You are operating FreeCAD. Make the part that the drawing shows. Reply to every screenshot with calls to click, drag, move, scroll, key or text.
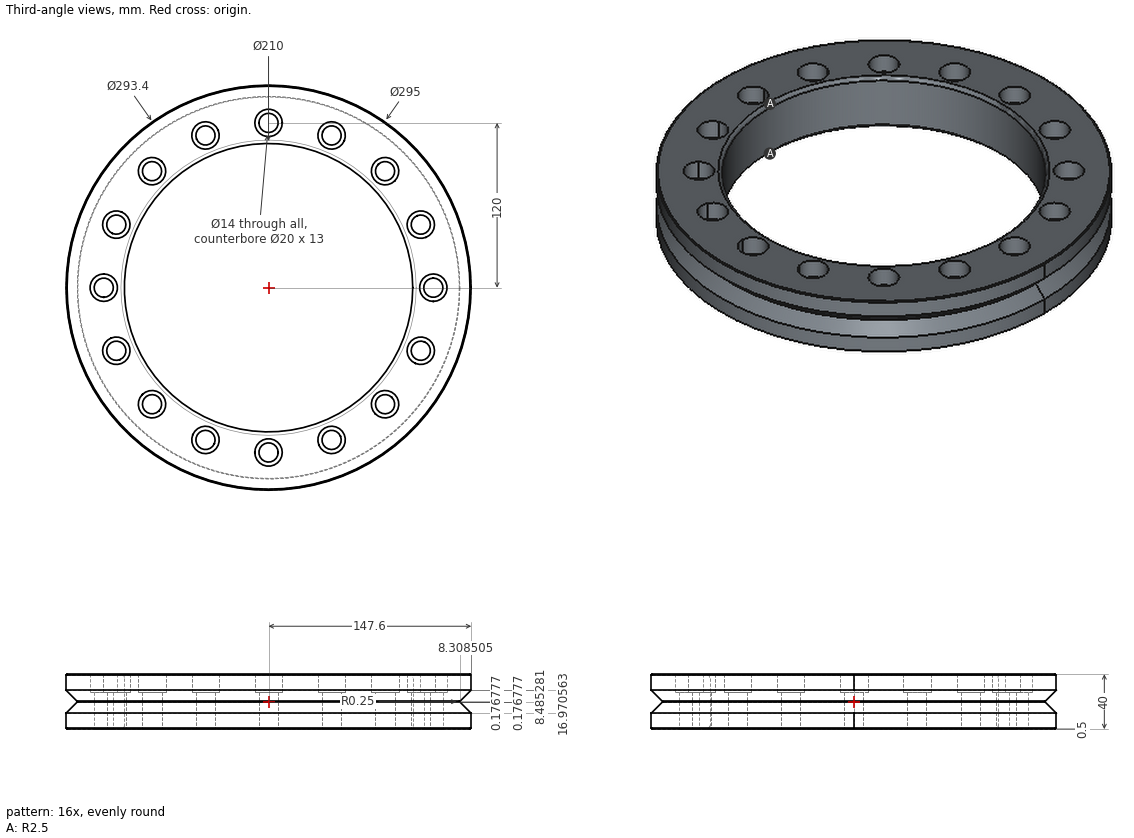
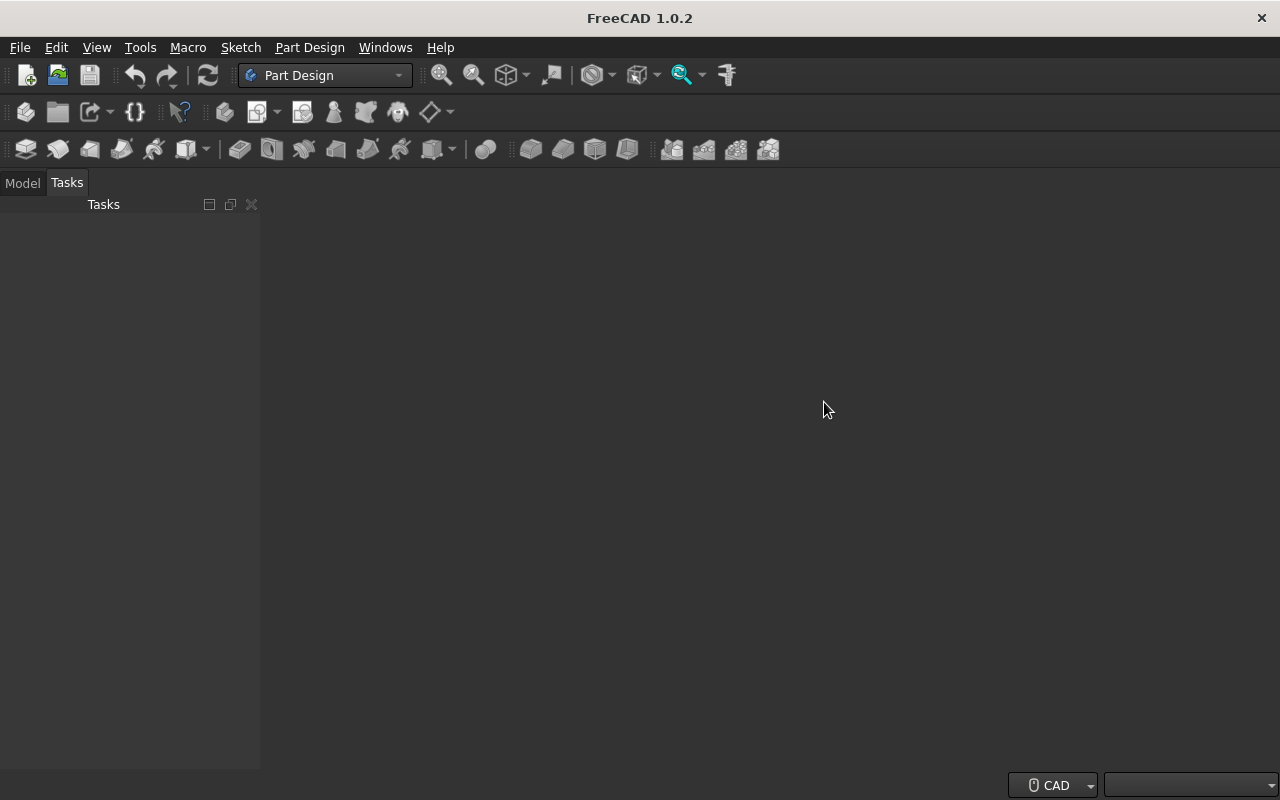
key(ctrl+n)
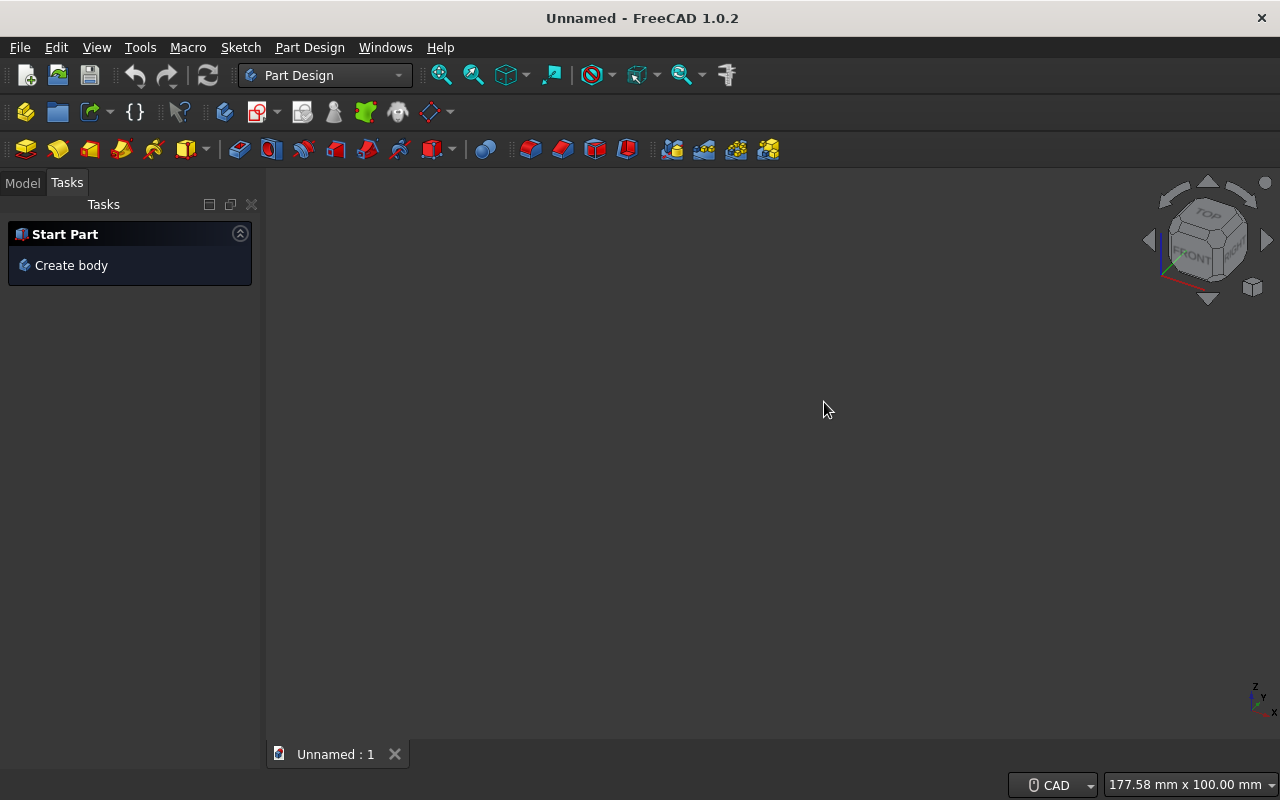
click(258, 112)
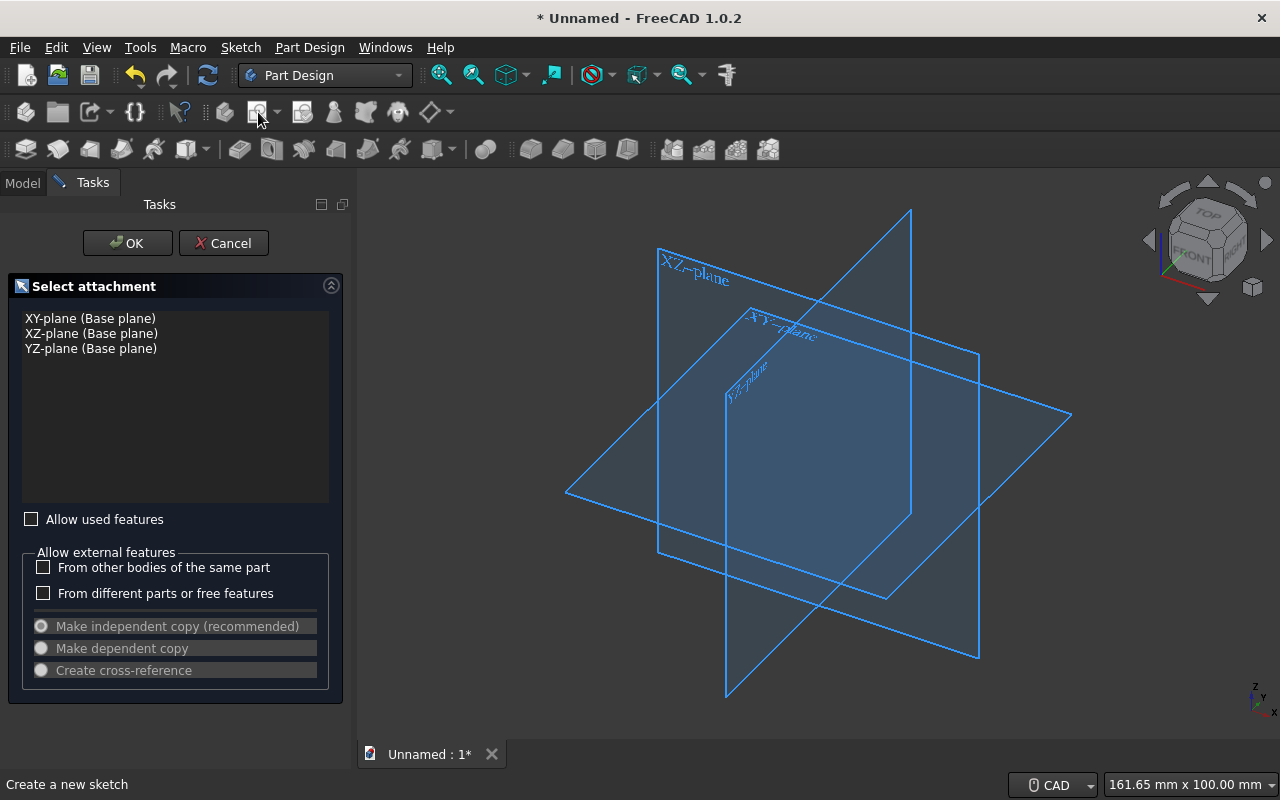
click(82, 318)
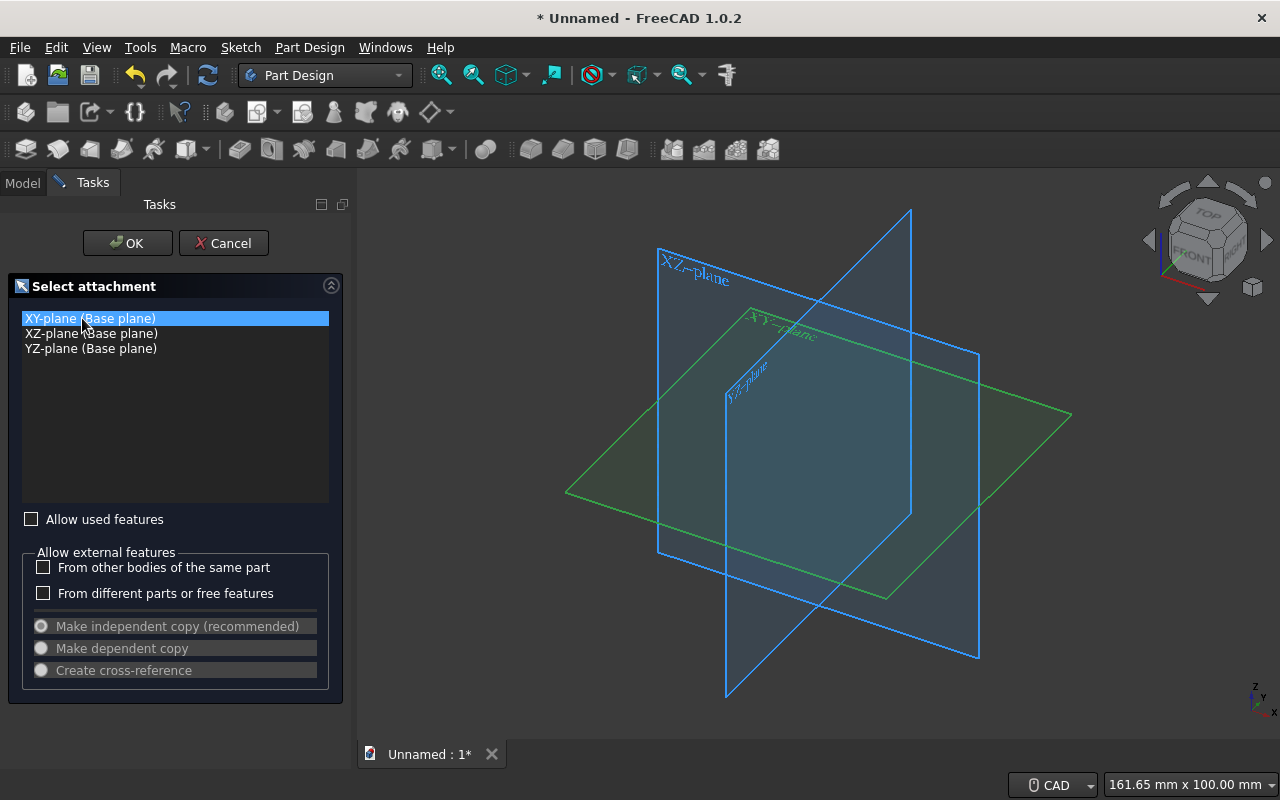
click(128, 243)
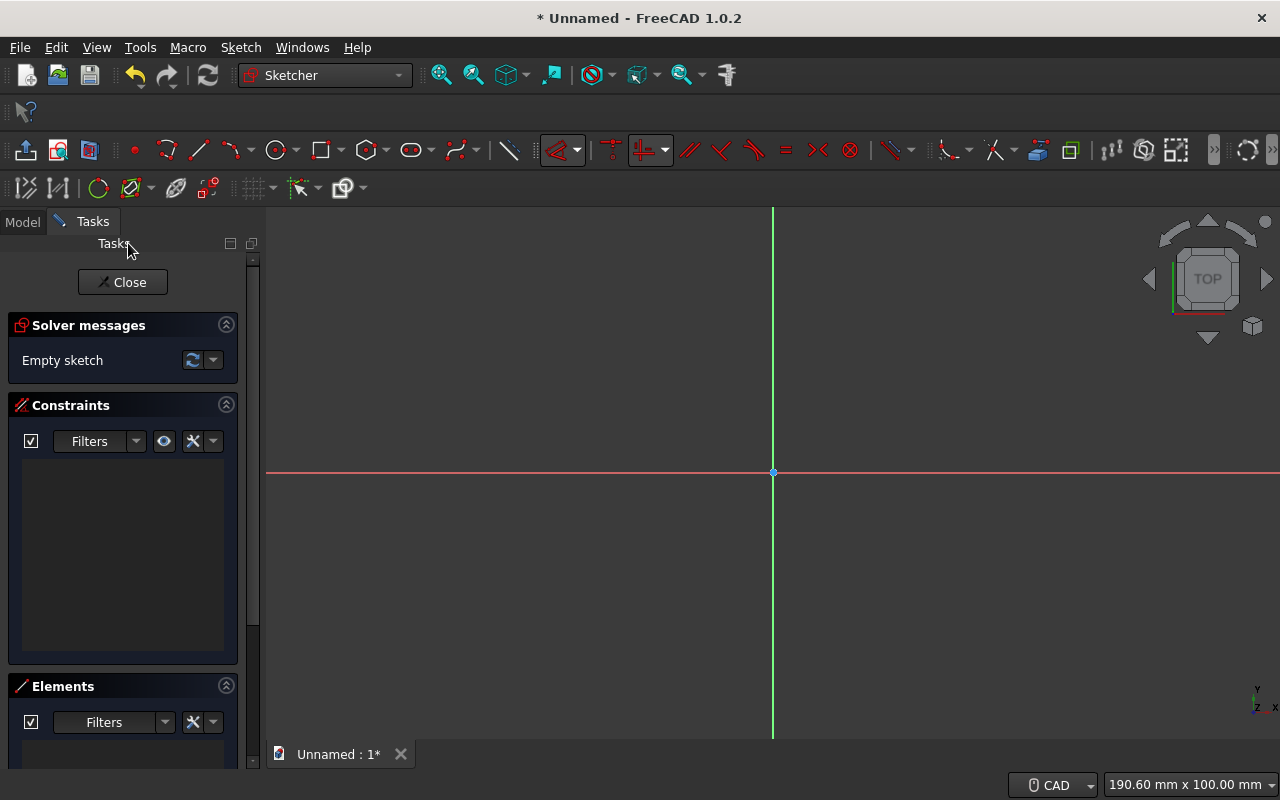
scroll(687, 473, down, 8)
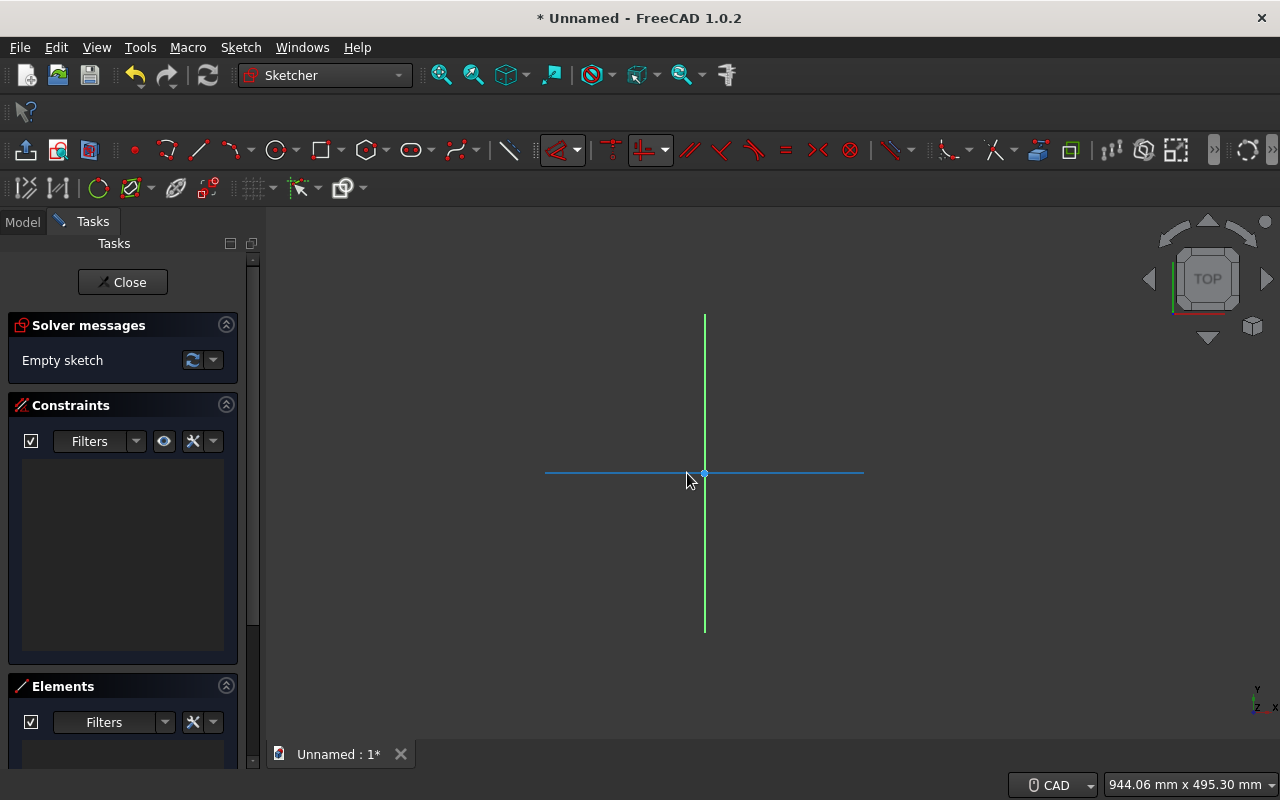
click(276, 150)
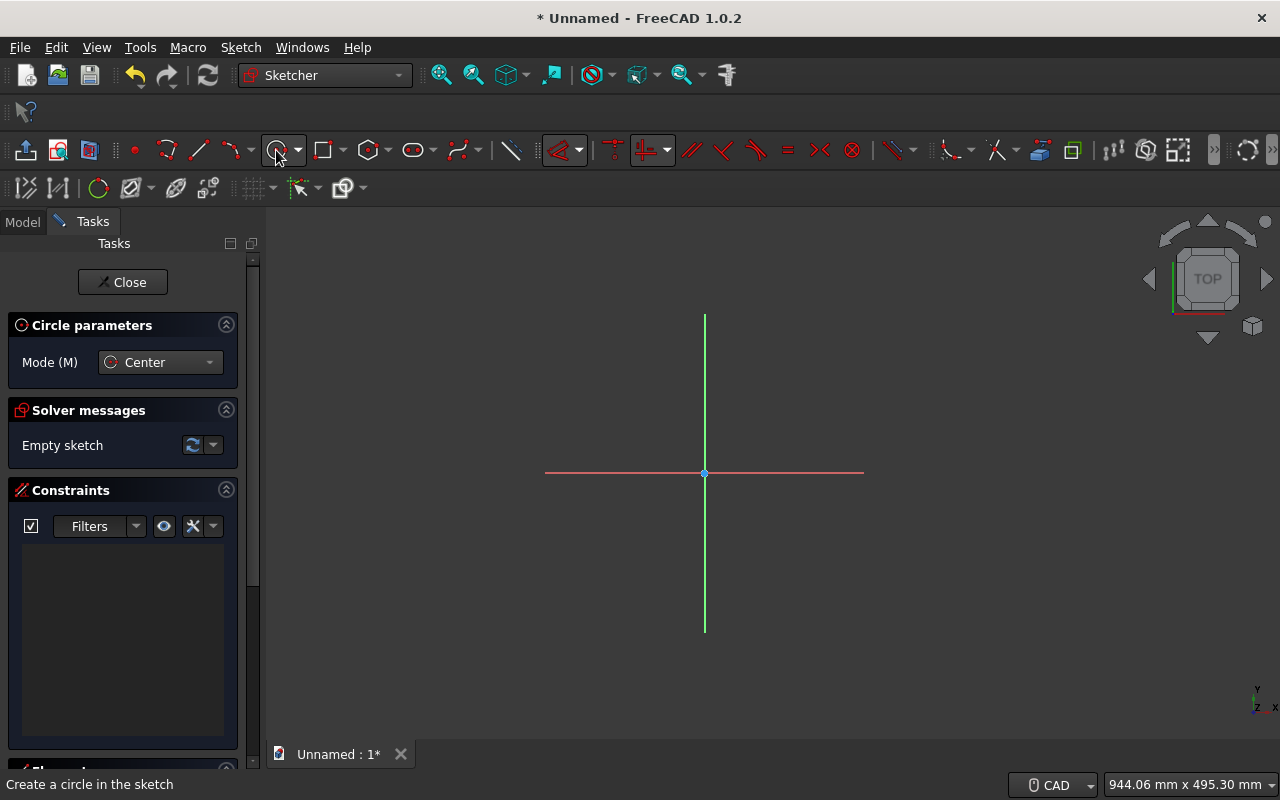
click(705, 473)
move(817, 361)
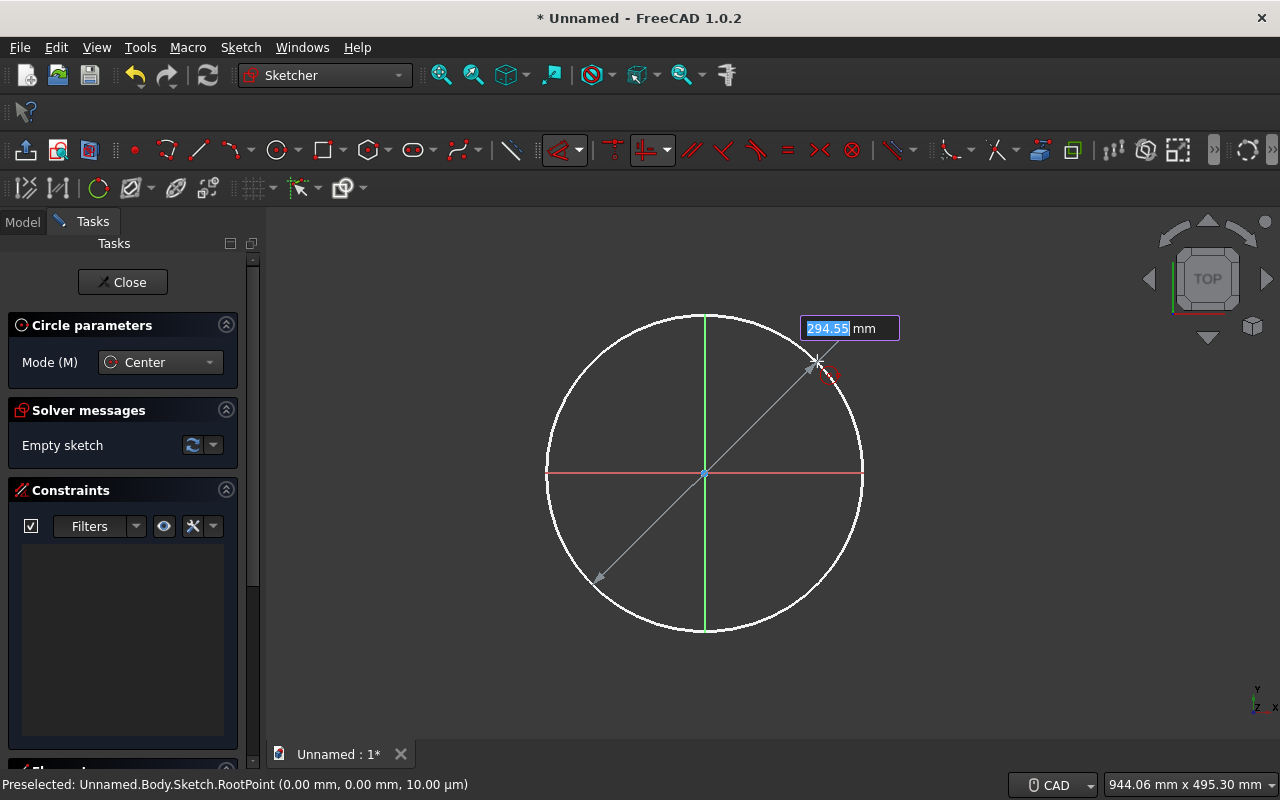
text(295)
key(Return)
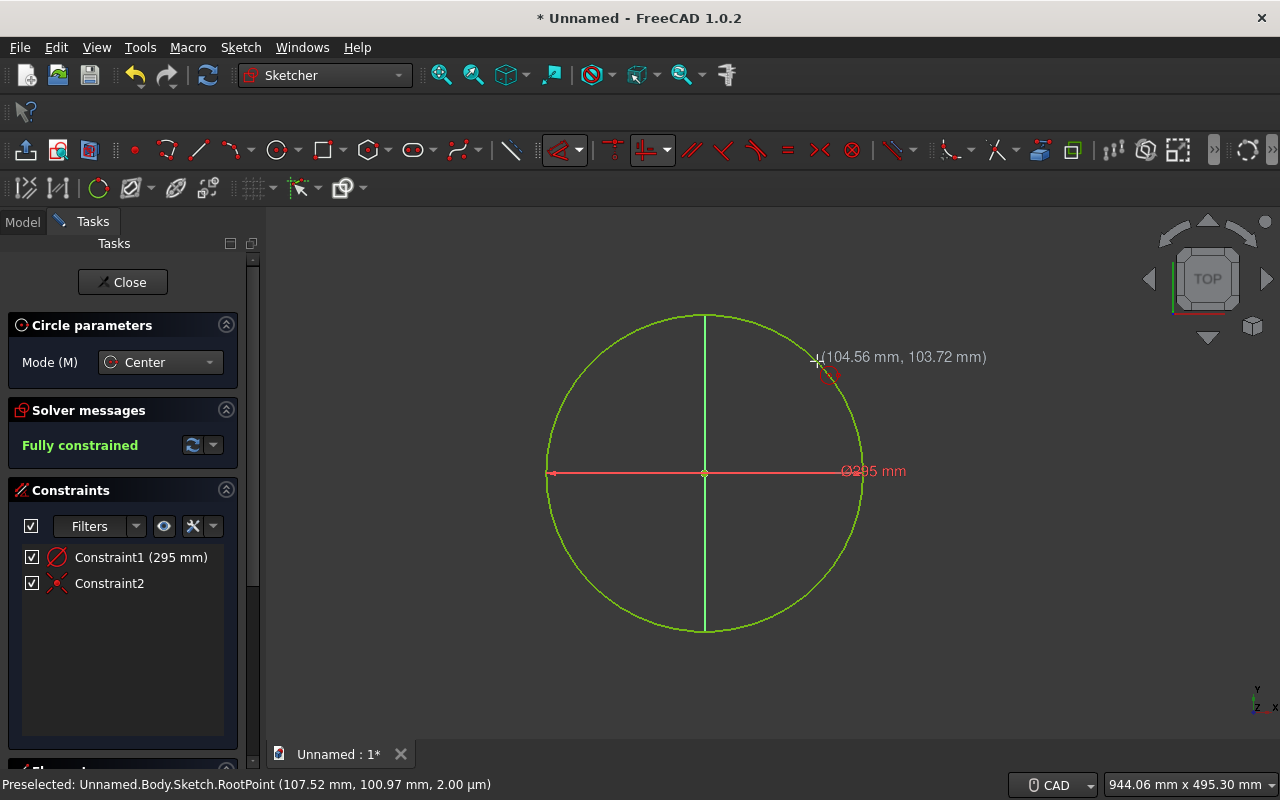
click(705, 473)
move(784, 394)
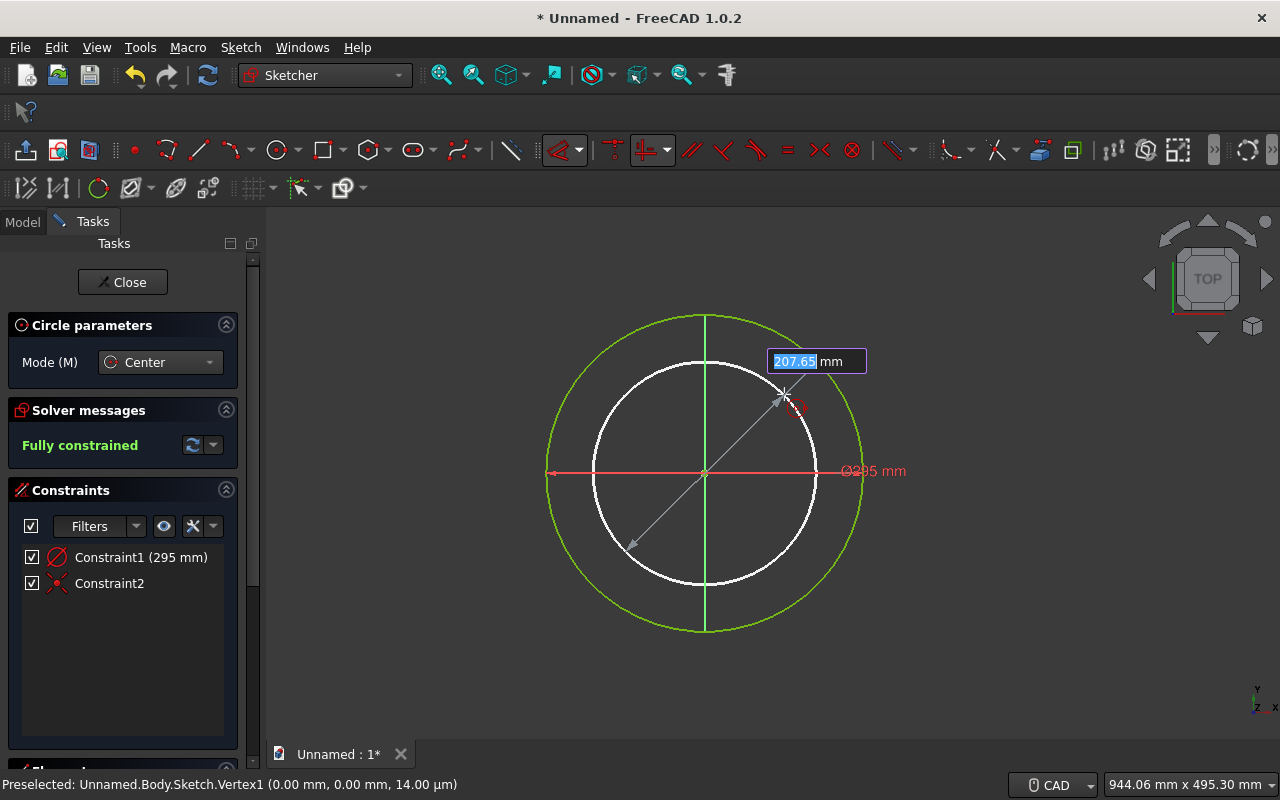
text(210)
key(Return)
key(Escape)